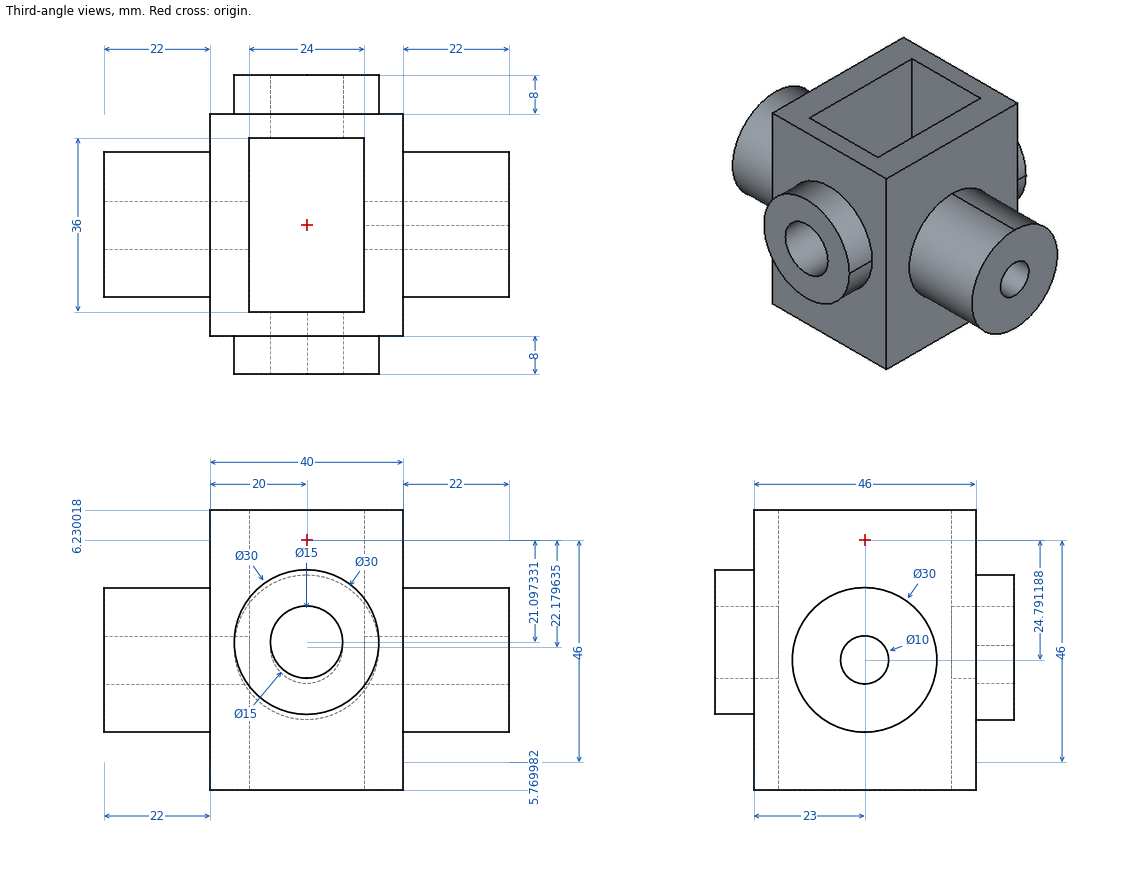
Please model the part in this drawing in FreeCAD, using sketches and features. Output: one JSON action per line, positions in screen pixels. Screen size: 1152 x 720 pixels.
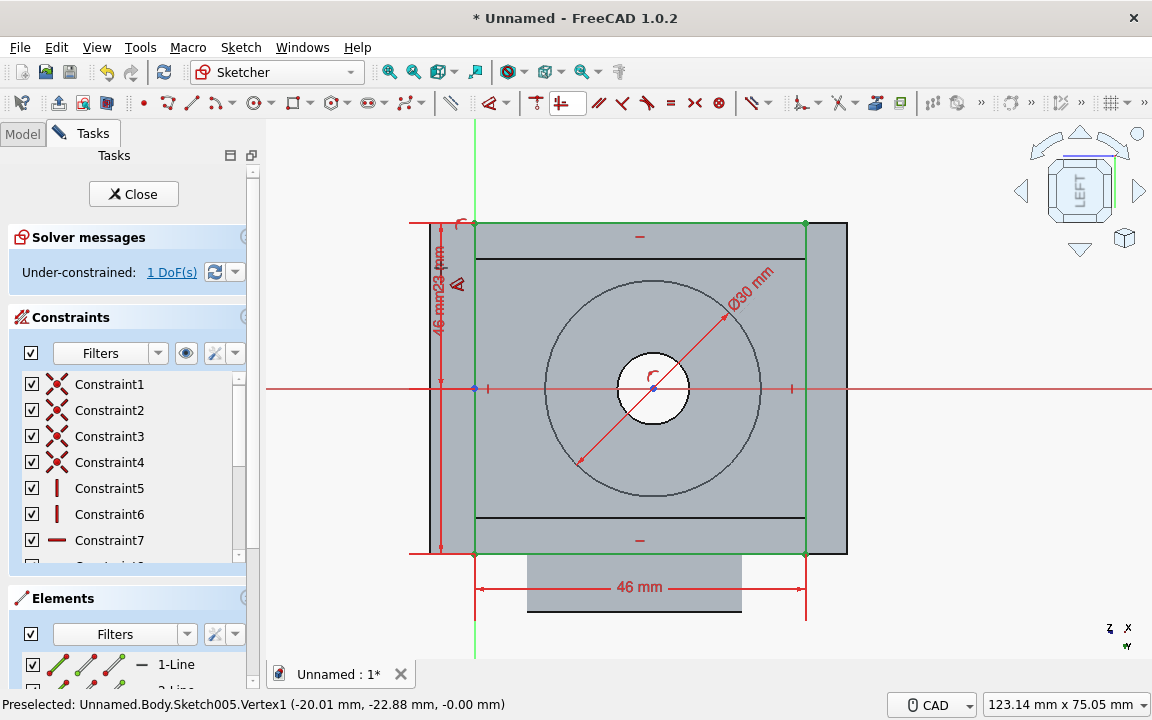
{"action": "left_click", "coordinate": [653, 389]}
{"action": "left_click", "coordinate": [523, 423]}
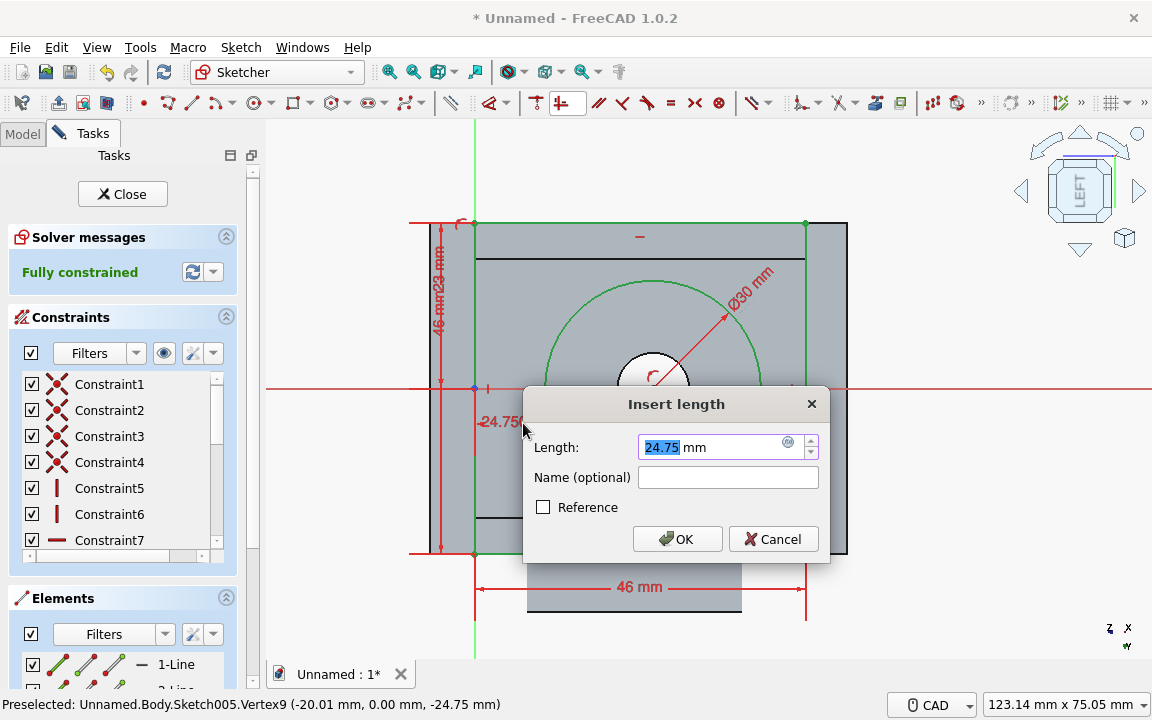
{"action": "type", "text": "24.791188"}
{"action": "key", "text": "Return"}
{"action": "key", "text": "Escape"}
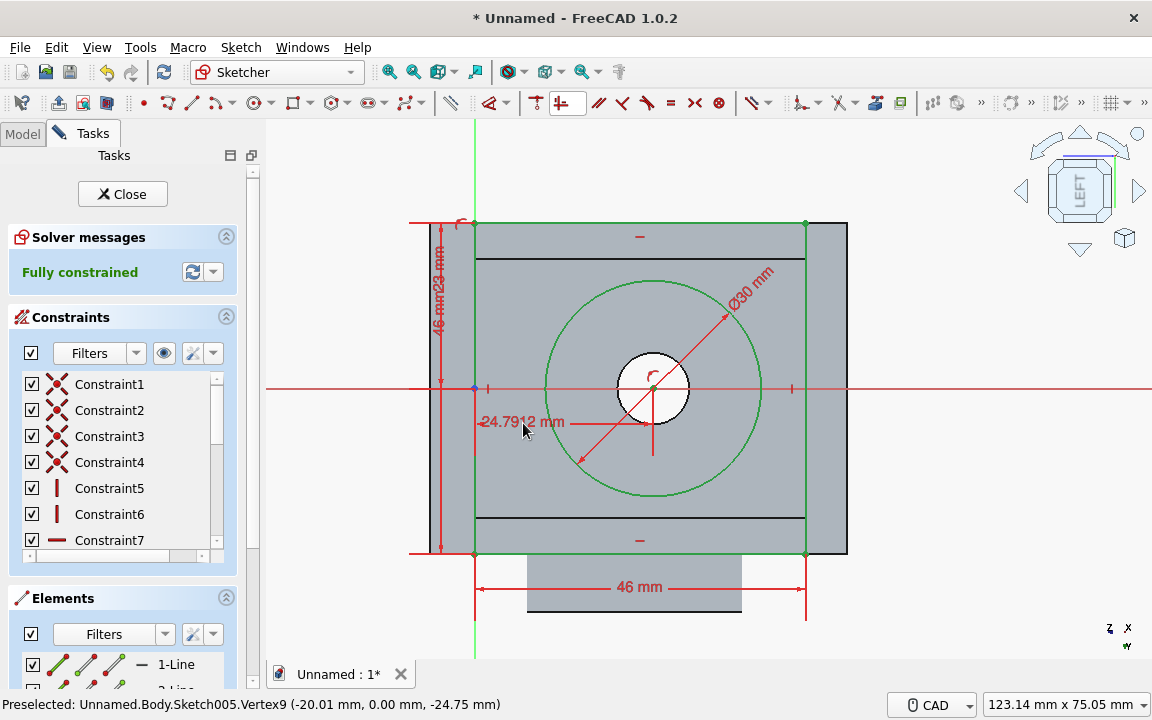
{"action": "left_click", "coordinate": [123, 194]}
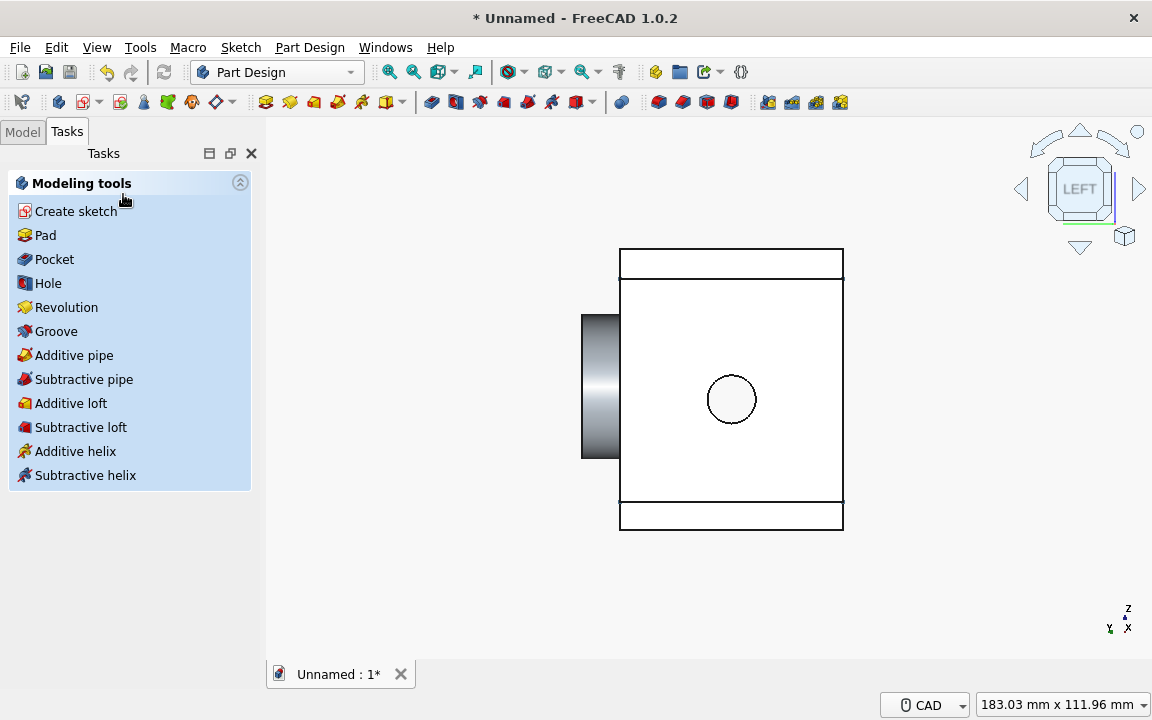
{"action": "left_click", "coordinate": [432, 102]}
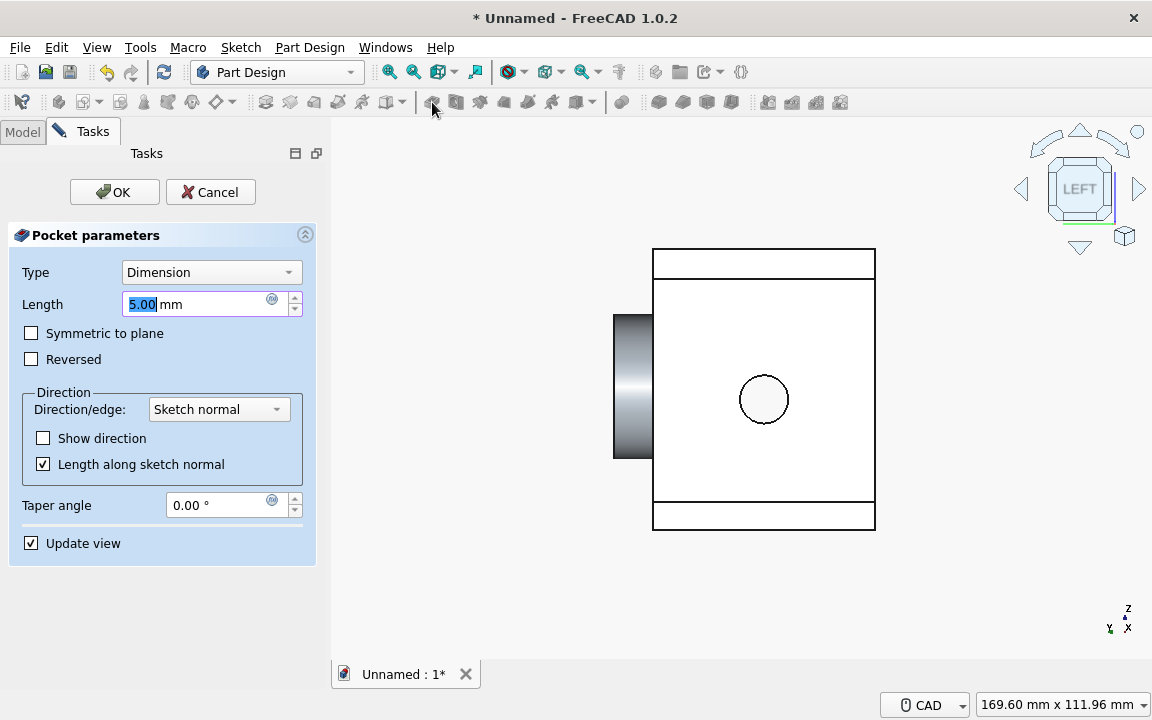
{"action": "type", "text": "22"}
{"action": "key", "text": "Tab"}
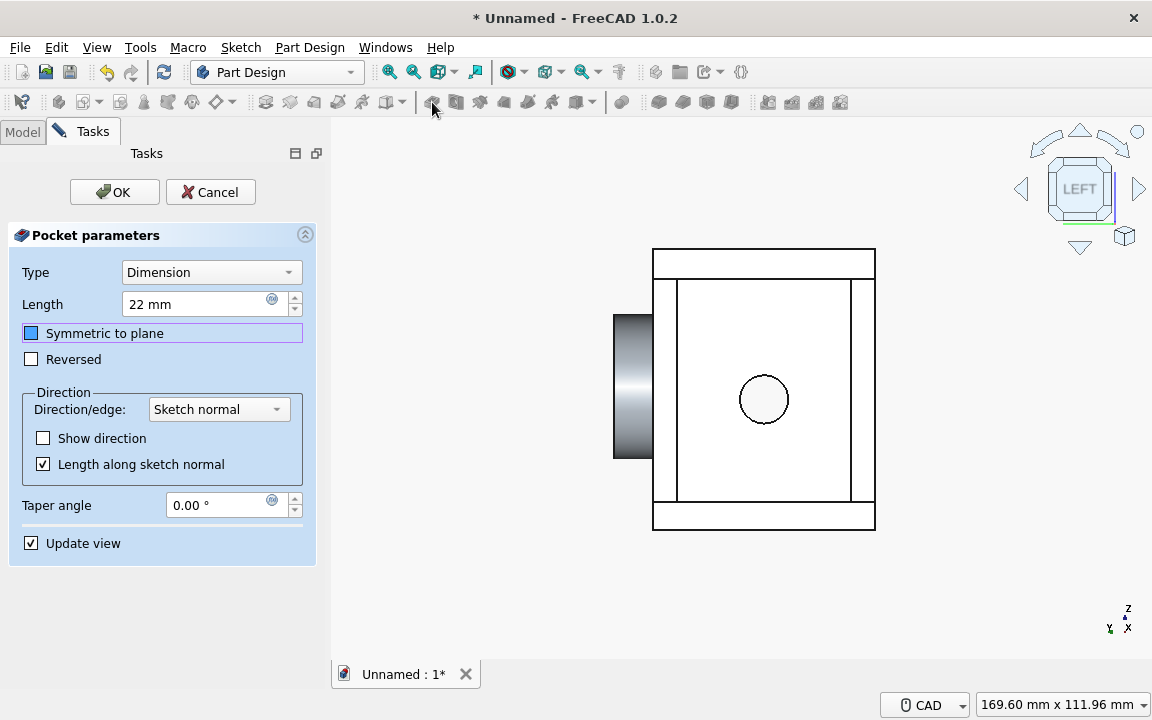
{"action": "left_click", "coordinate": [30, 359]}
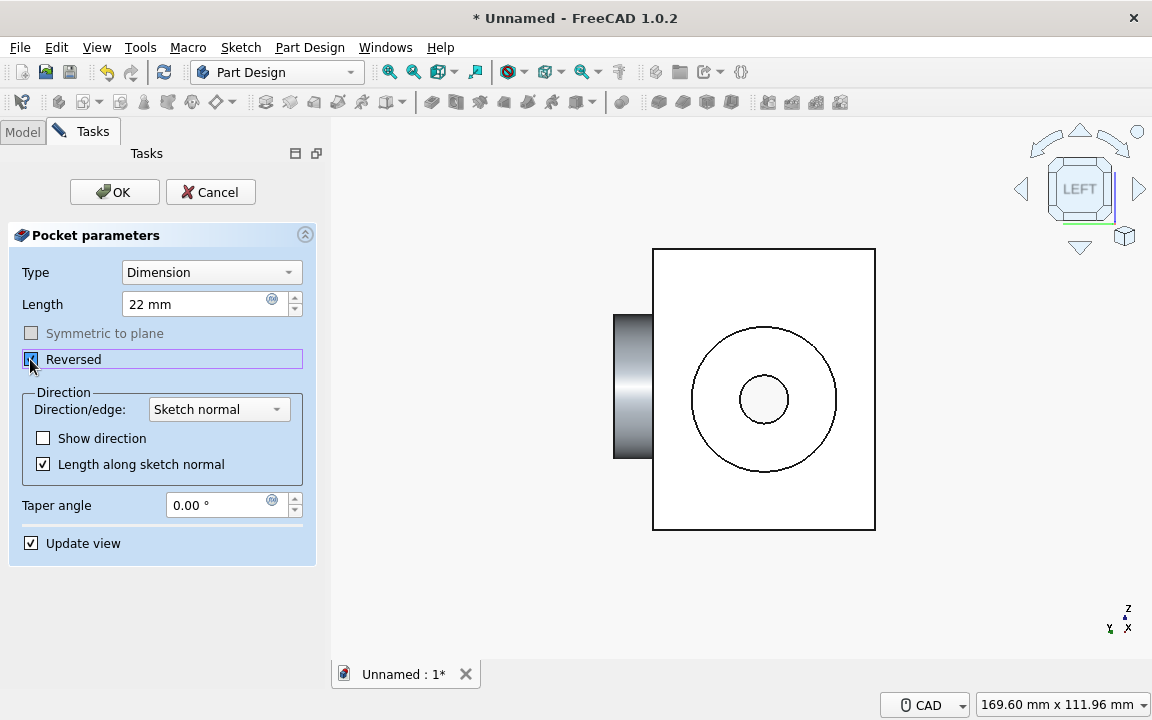
{"action": "left_click", "coordinate": [115, 192]}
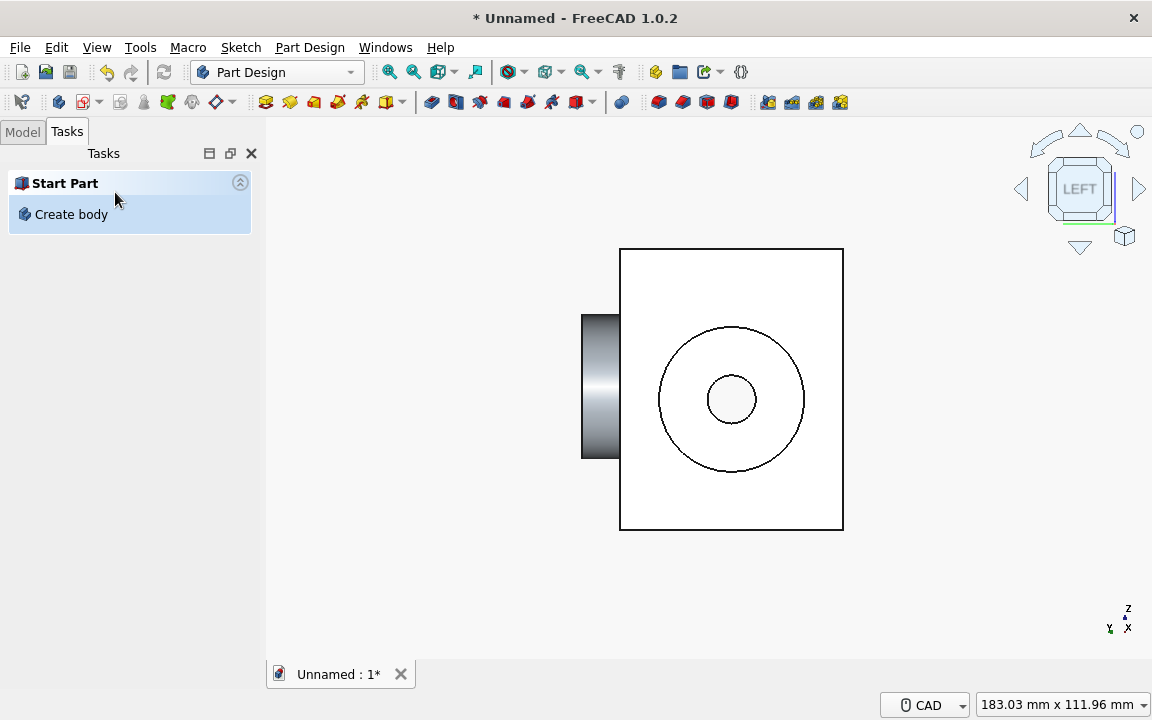
{"action": "key", "text": "0"}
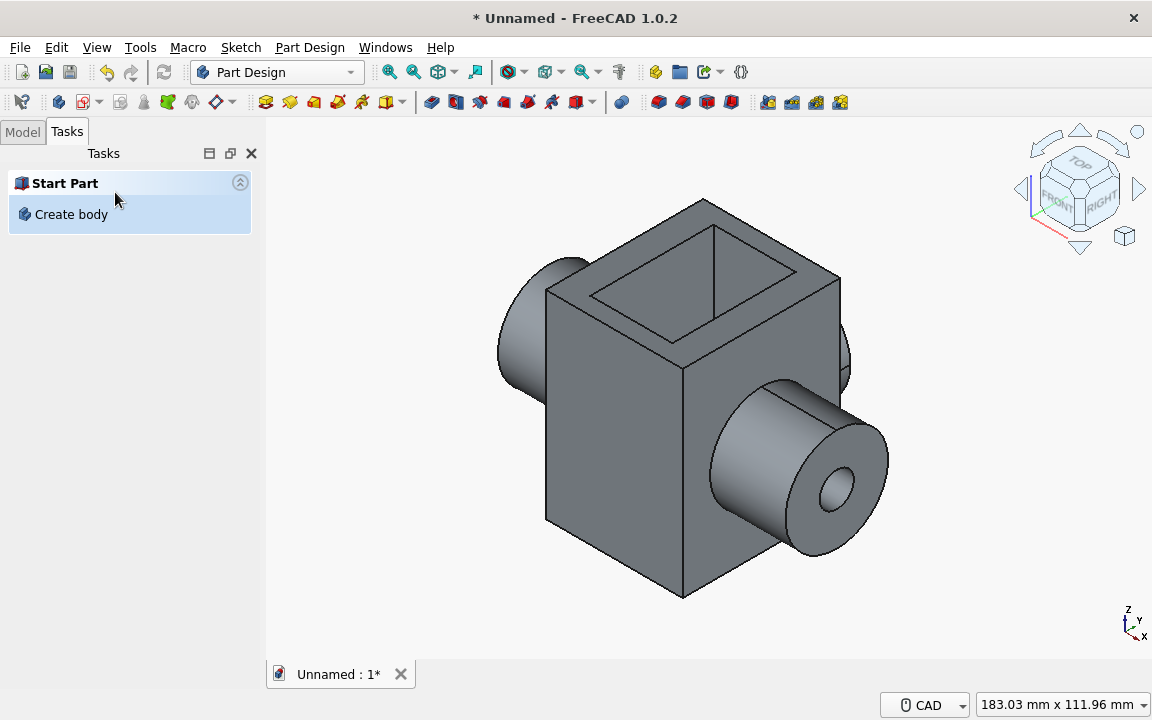
{"action": "left_click", "coordinate": [614, 410]}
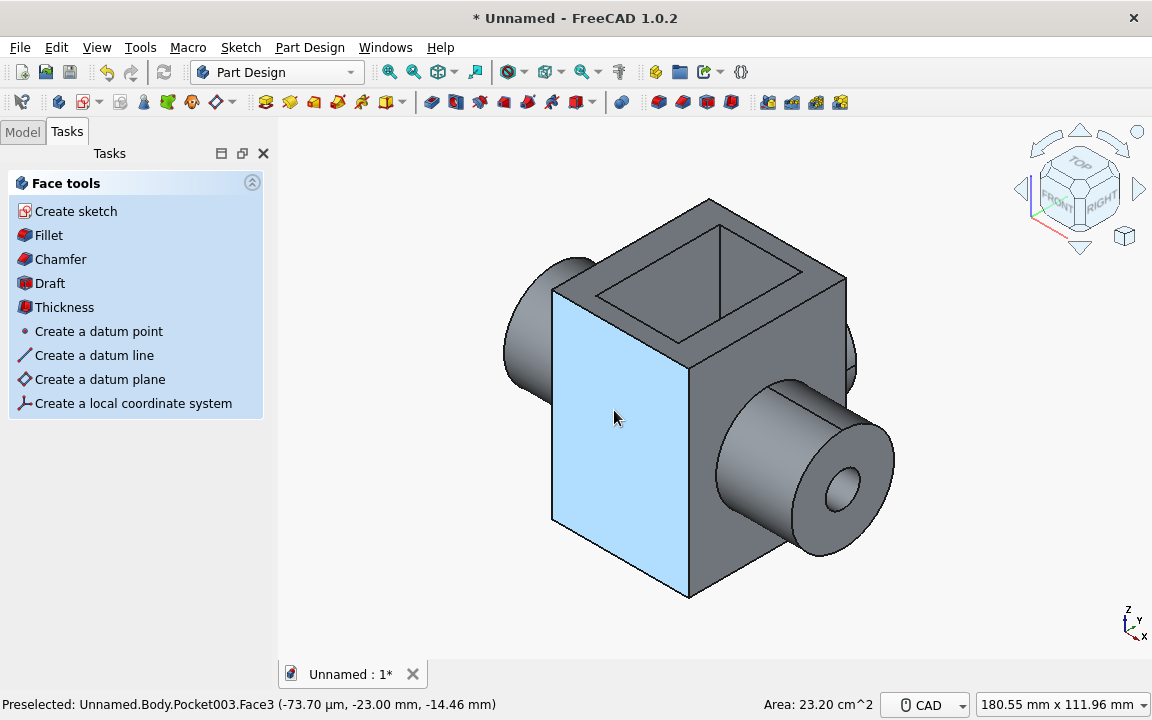
{"action": "left_click", "coordinate": [84, 102]}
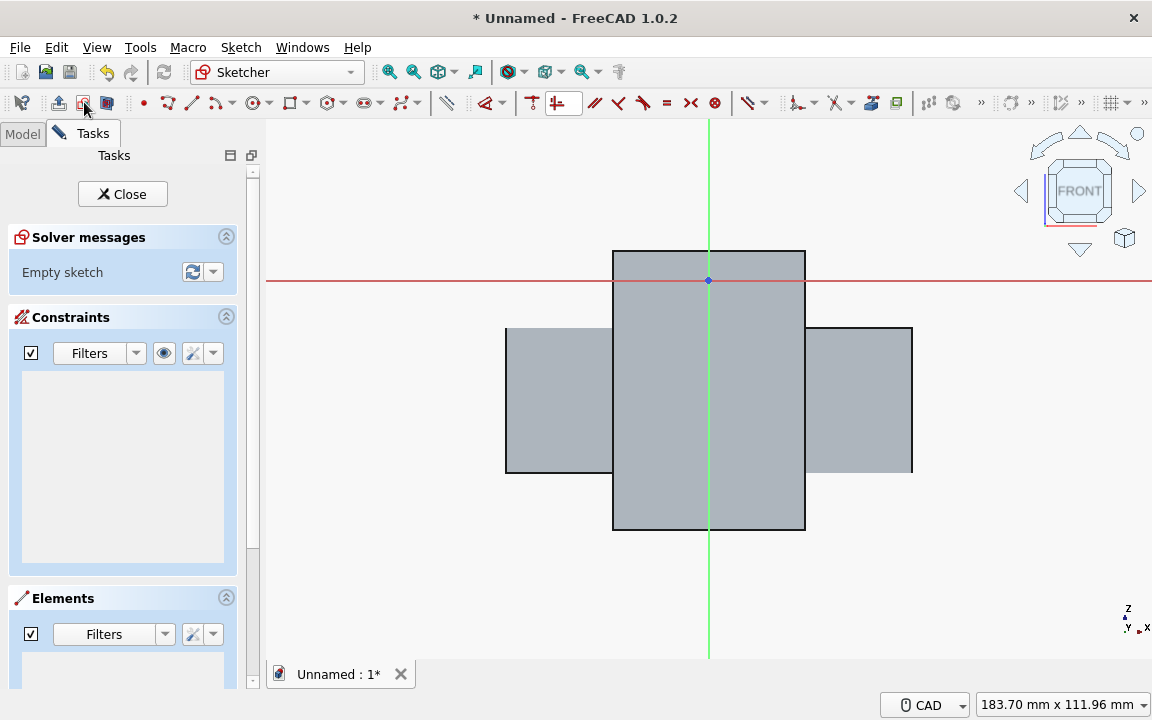
{"action": "scroll", "coordinate": [792, 342], "scroll_direction": "up", "scroll_amount": 3}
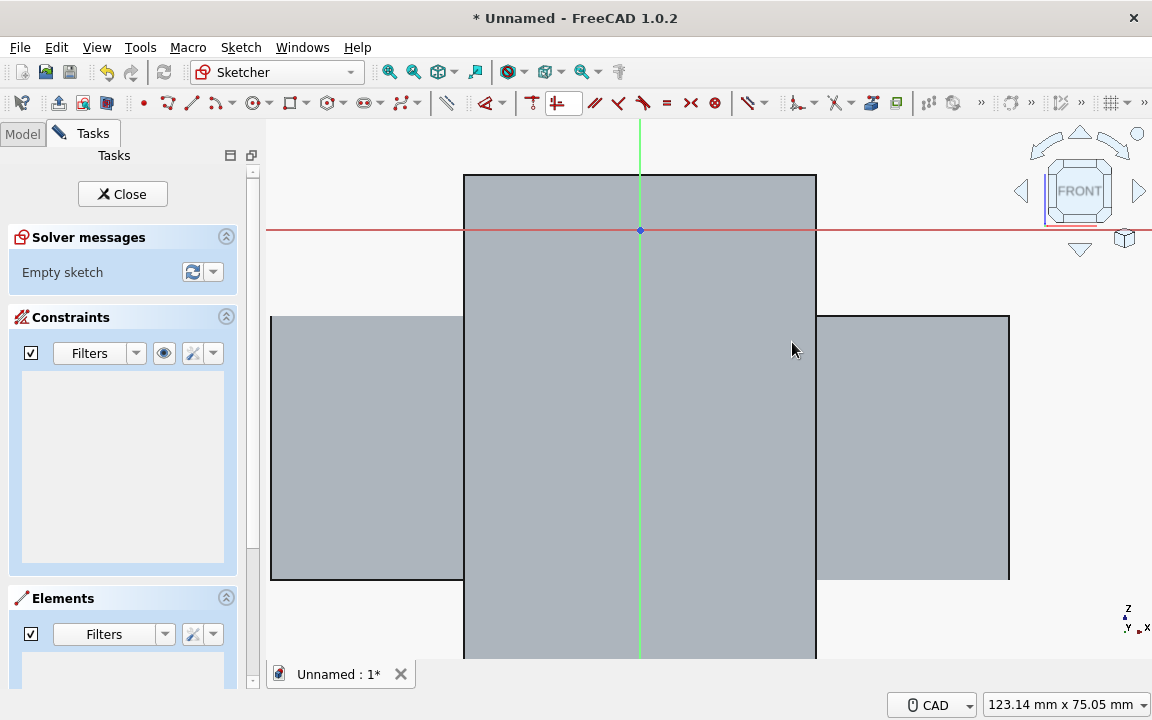
{"action": "left_click", "coordinate": [254, 104]}